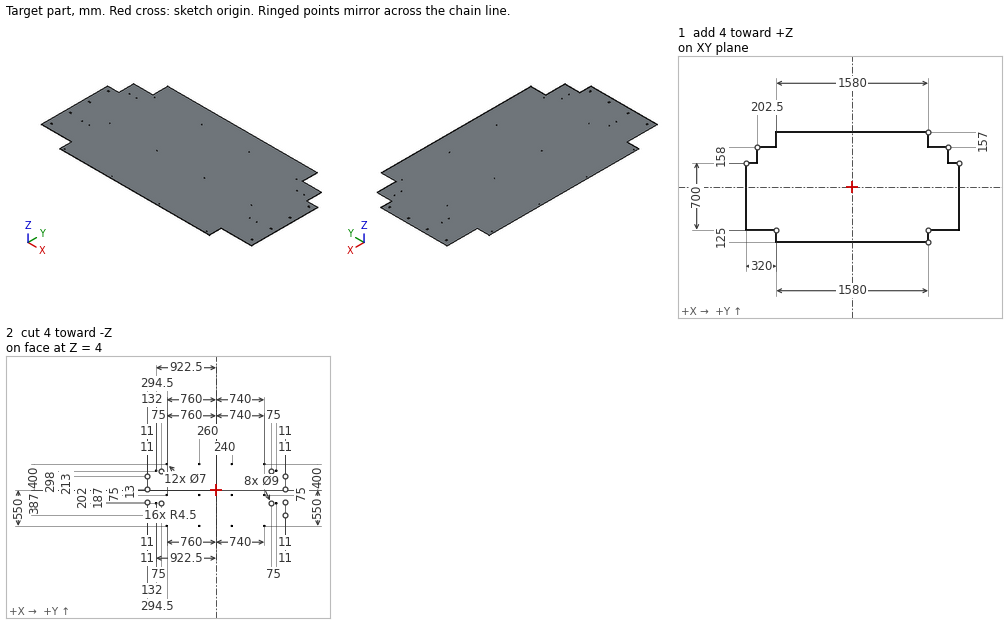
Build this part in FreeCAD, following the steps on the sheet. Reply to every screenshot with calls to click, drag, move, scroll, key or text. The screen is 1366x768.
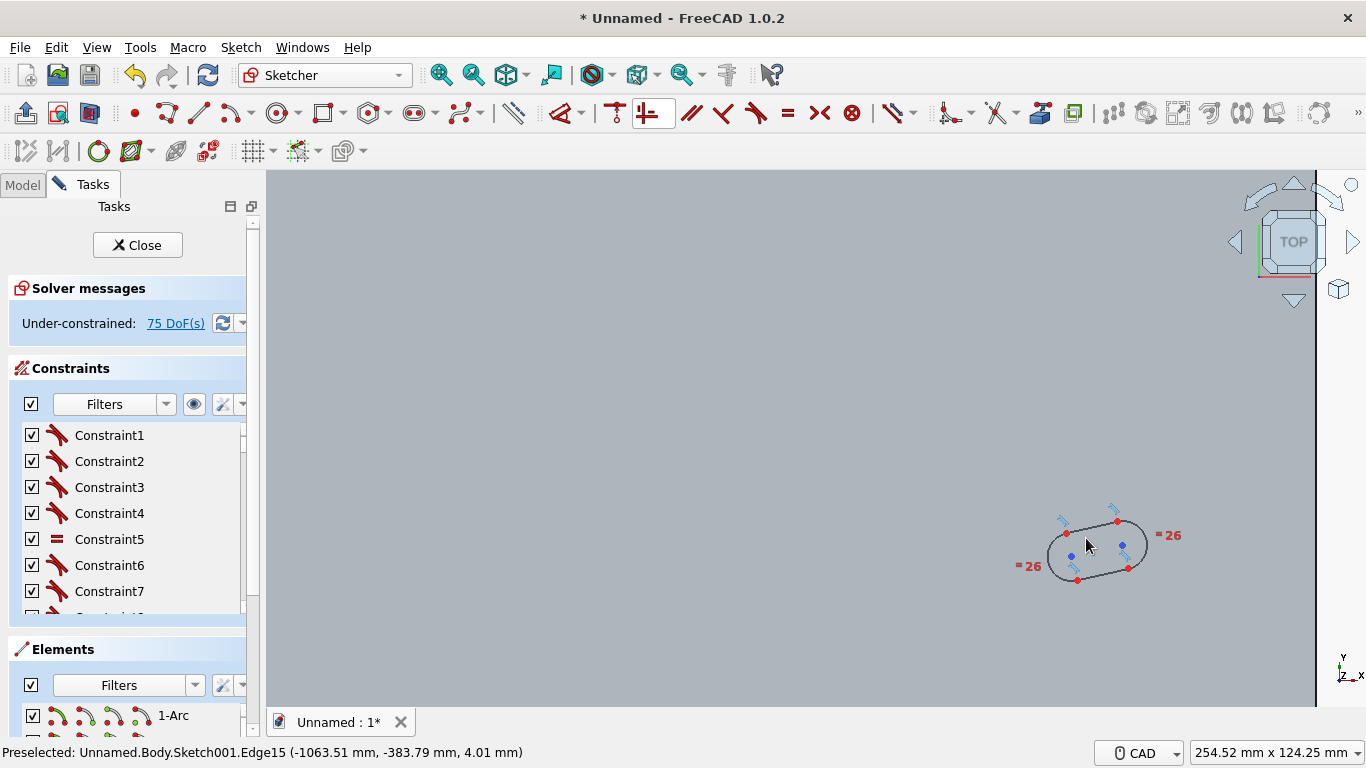
click(1082, 530)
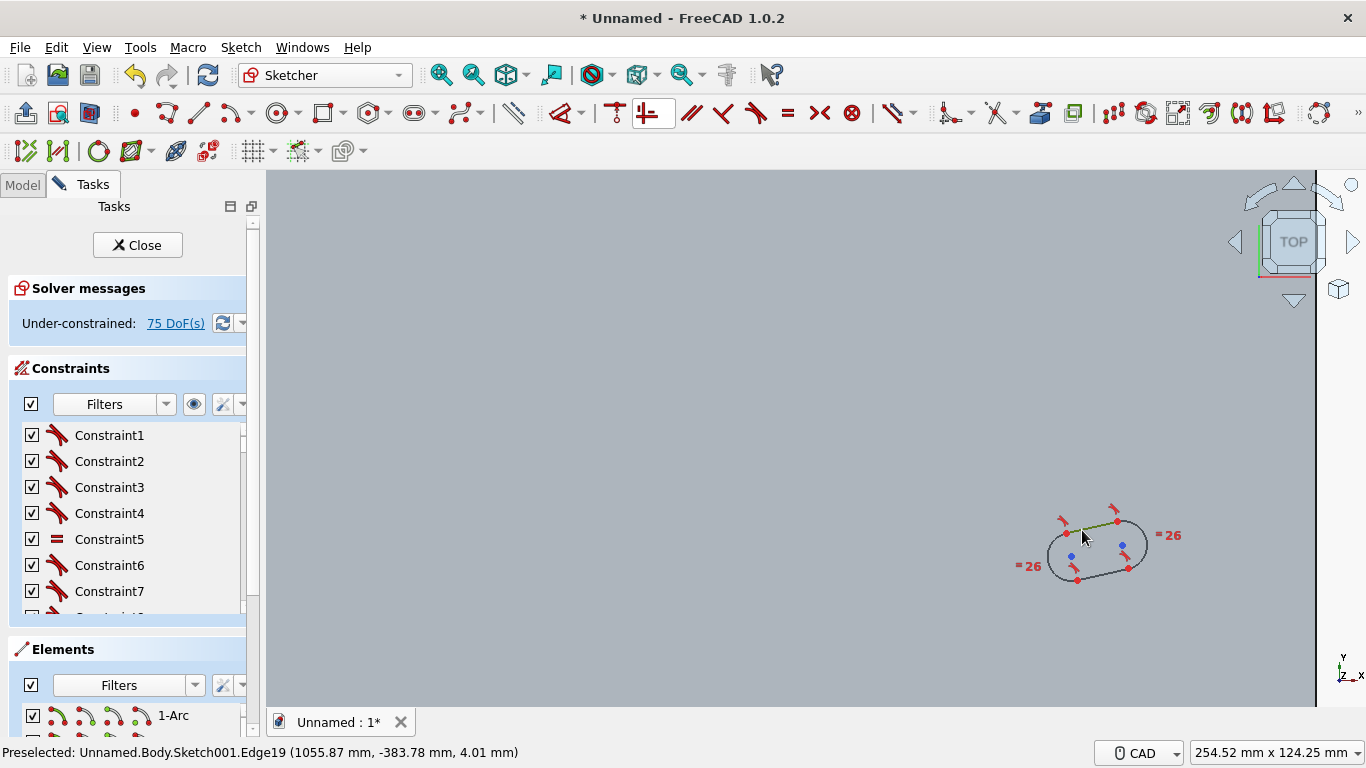
click(670, 114)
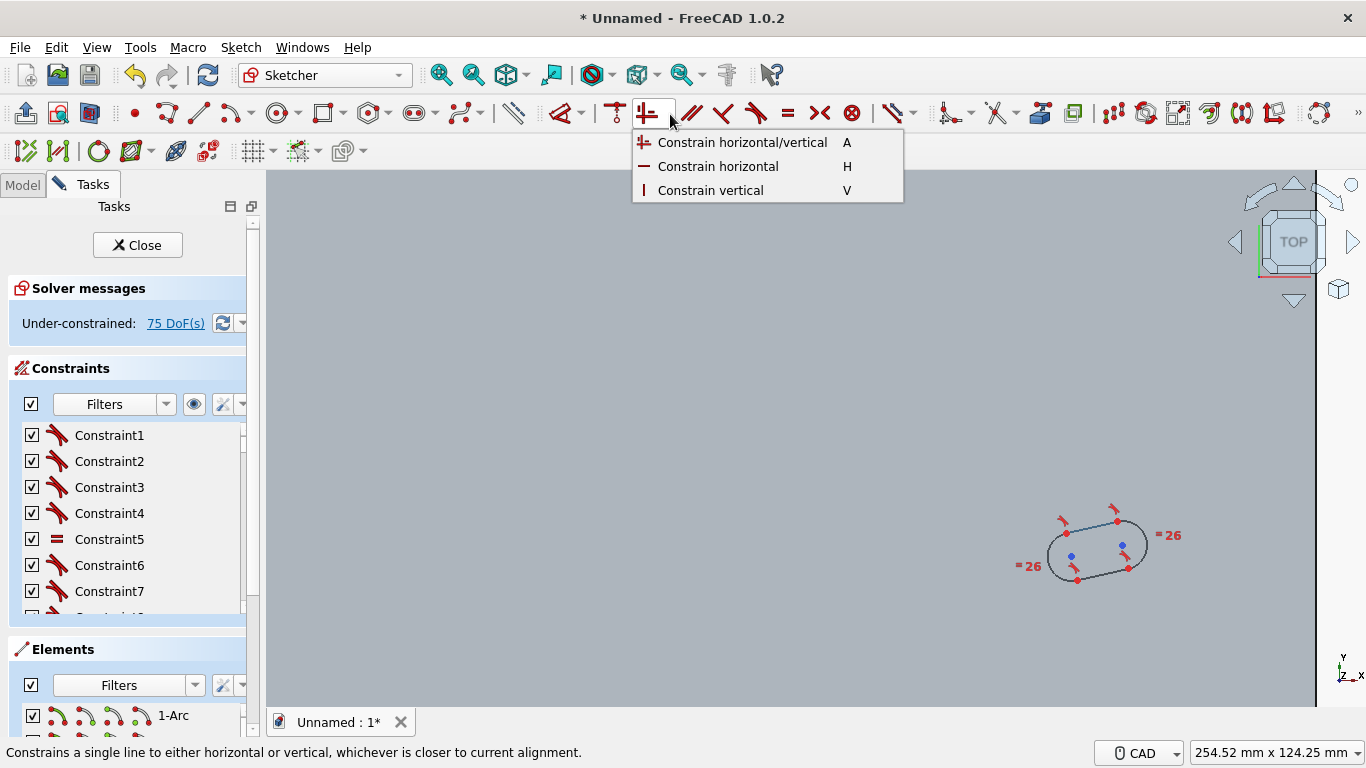
click(768, 166)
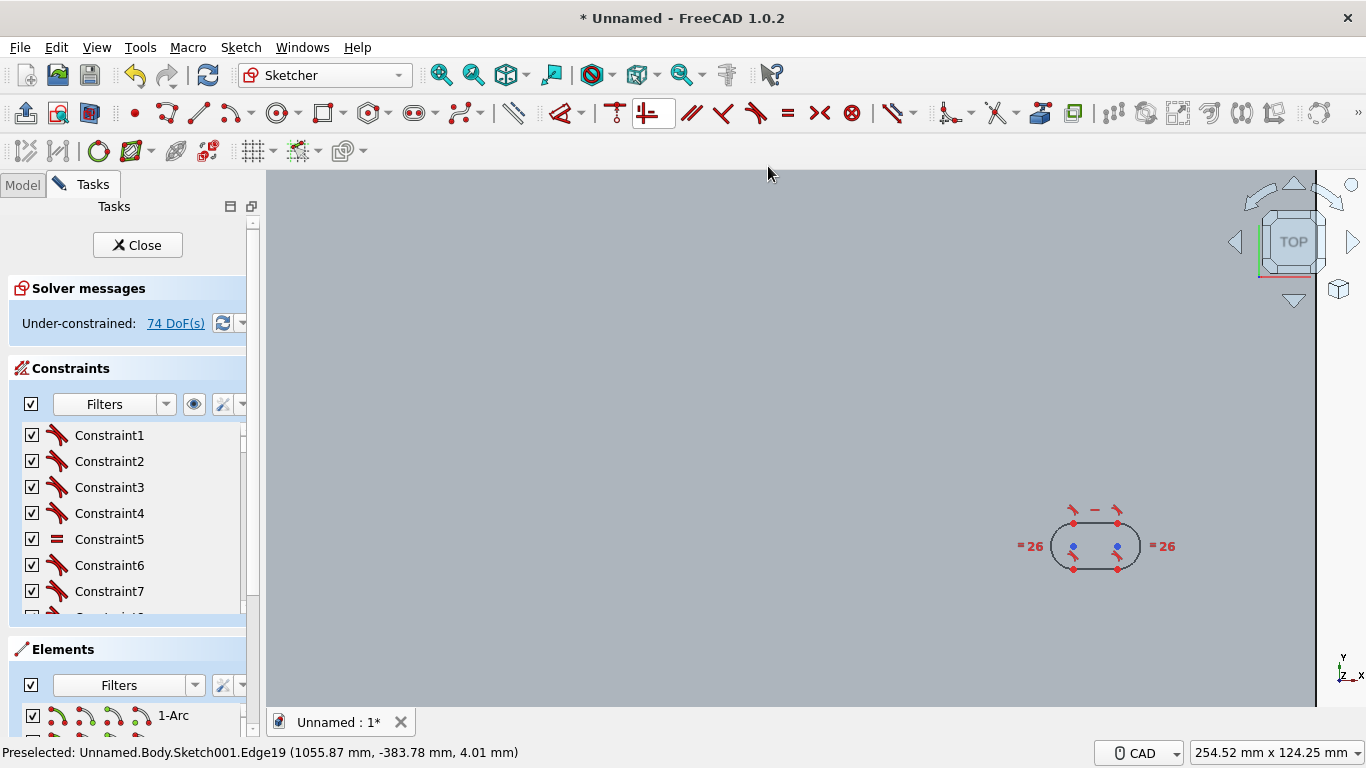
scroll(1087, 538, down, 13)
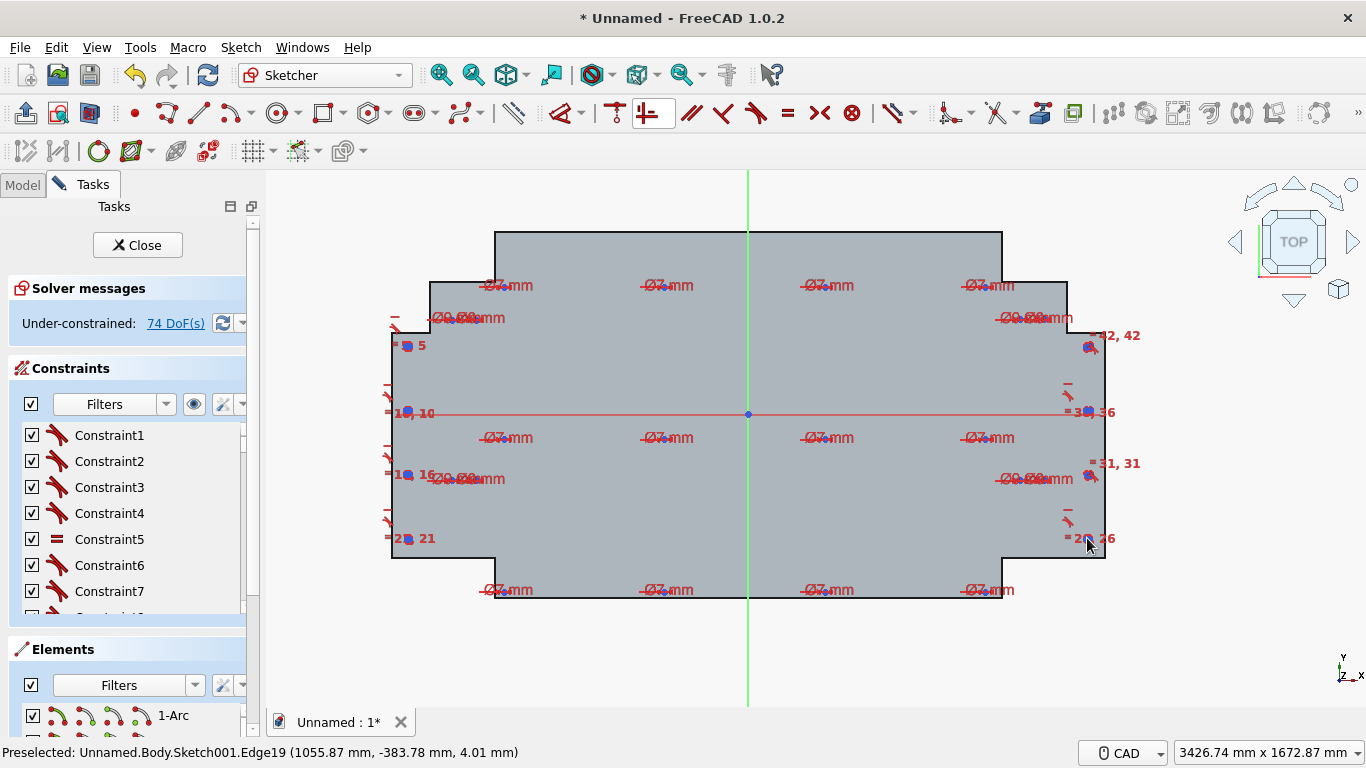
scroll(1088, 474, up, 13)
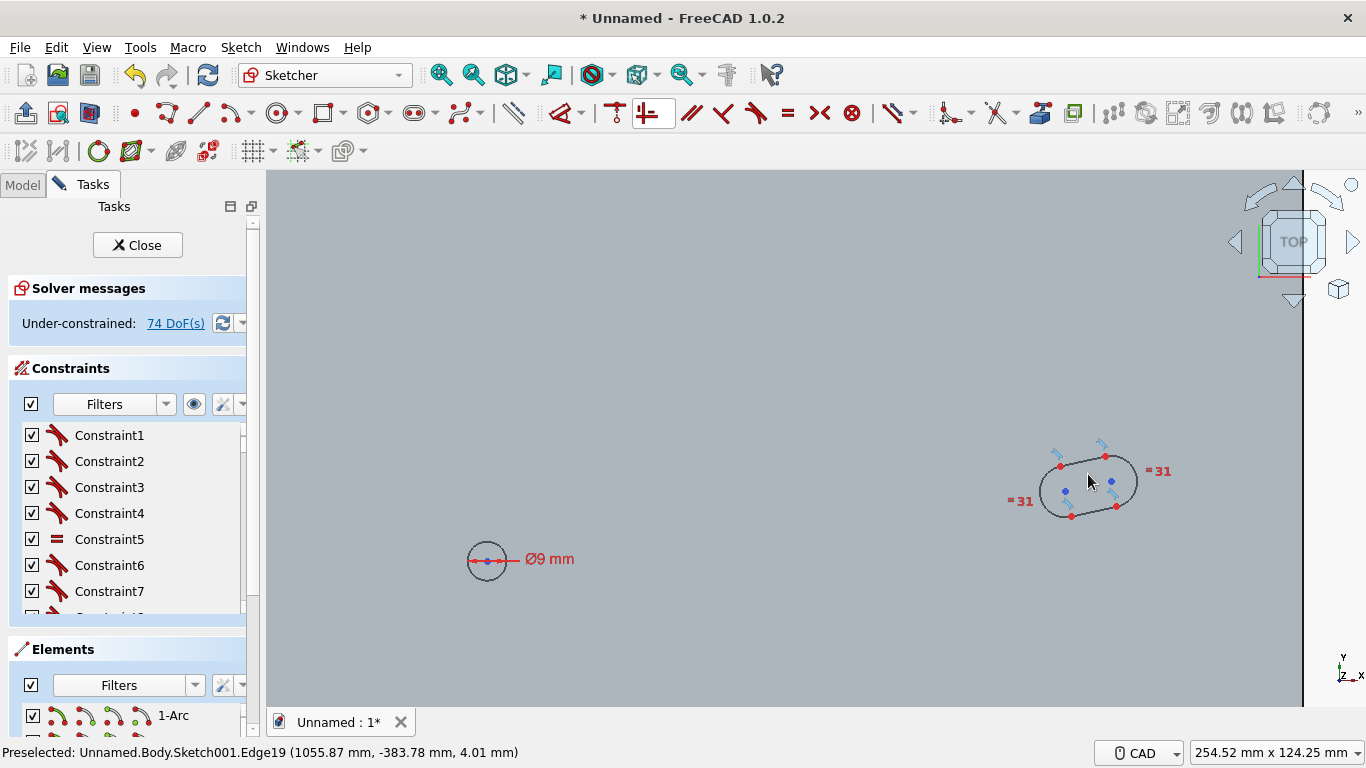
click(1074, 464)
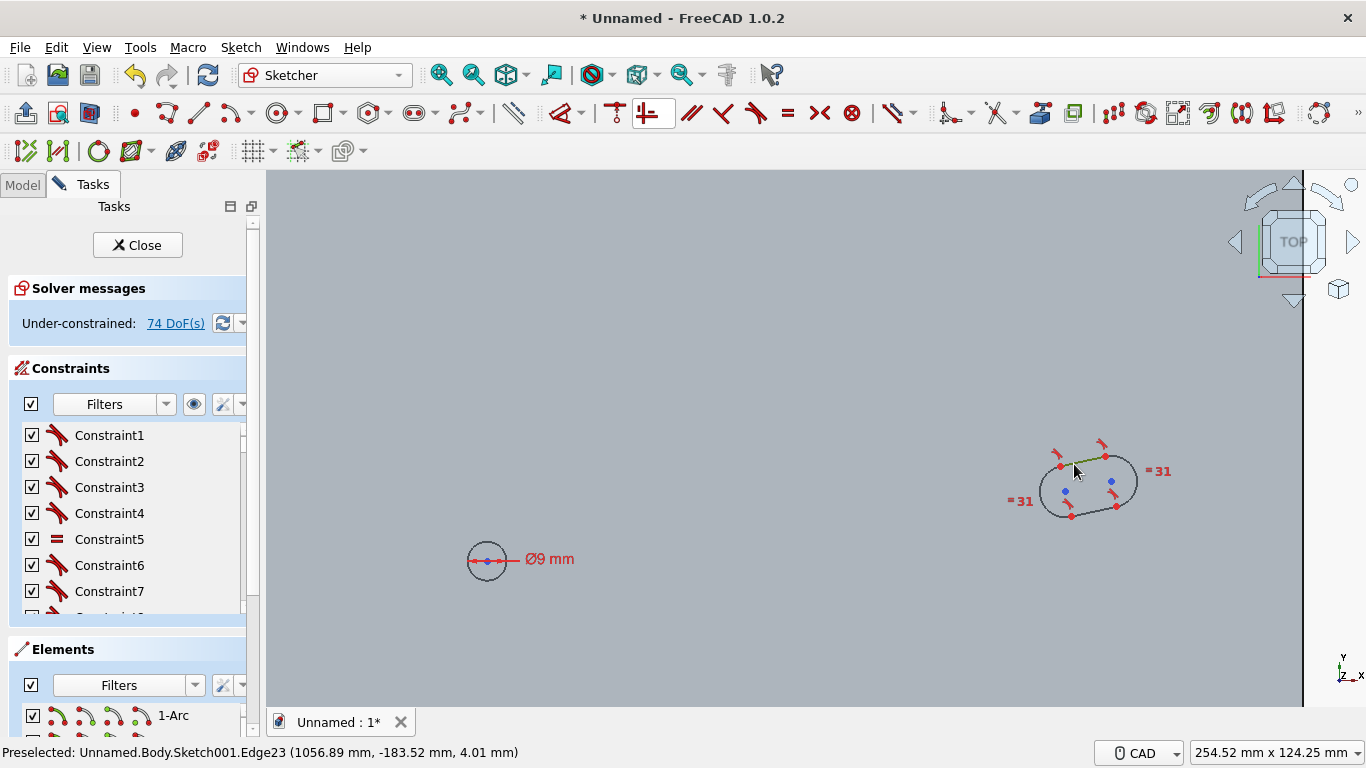
key(h)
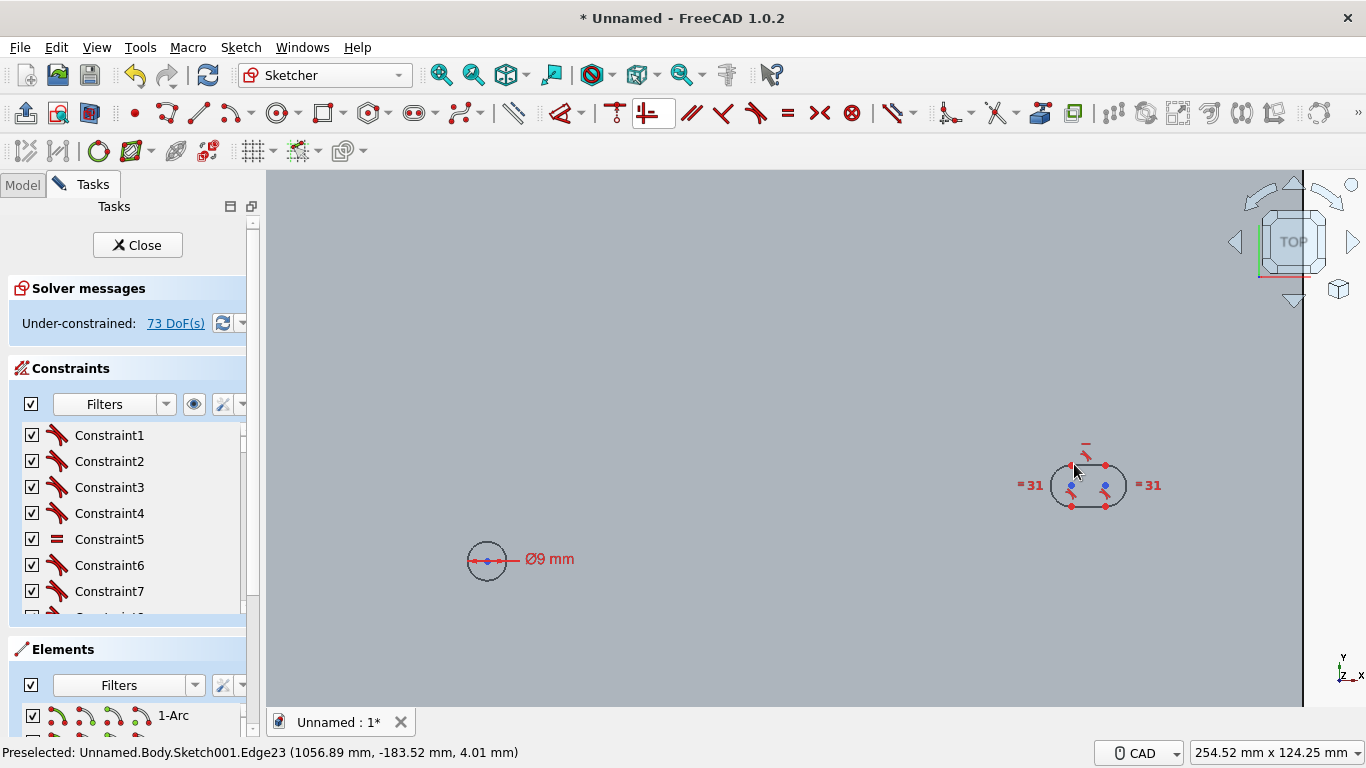
scroll(1088, 474, down, 13)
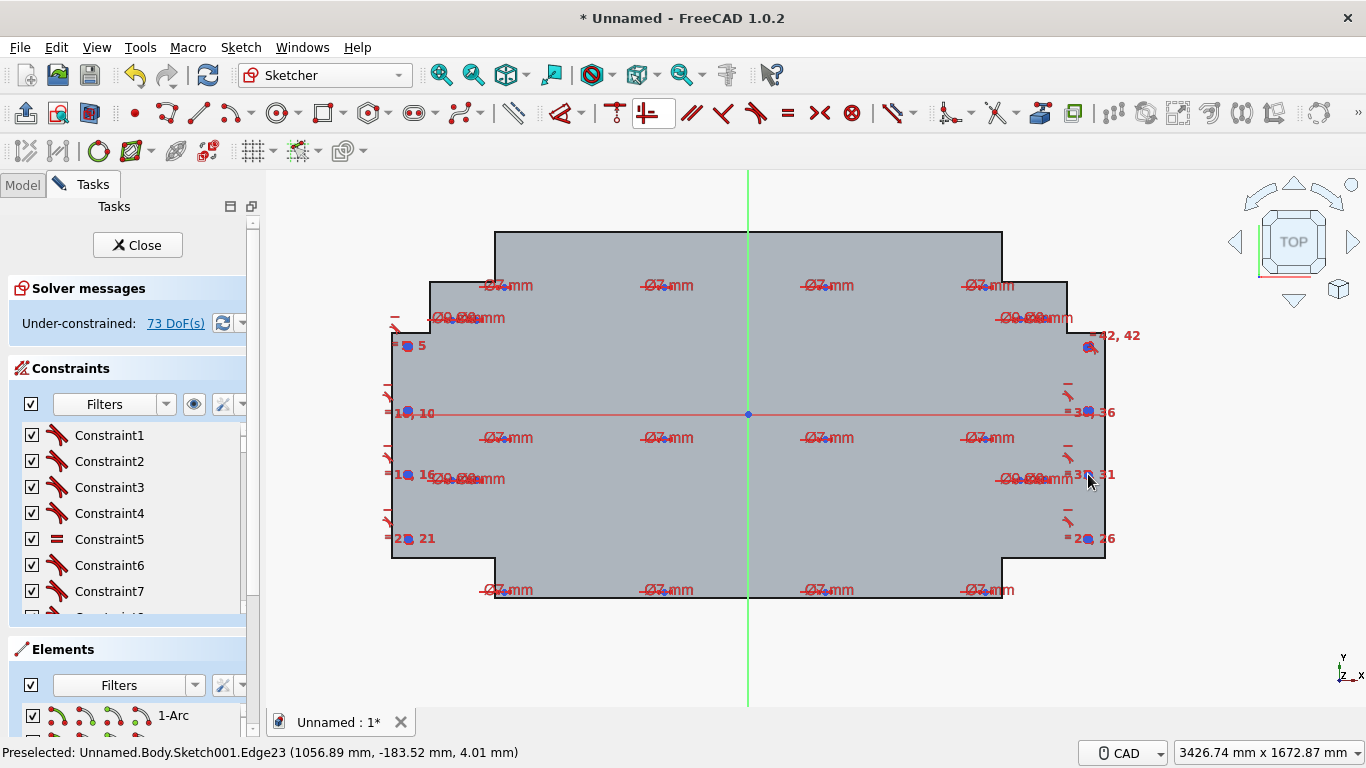
scroll(1087, 345, up, 13)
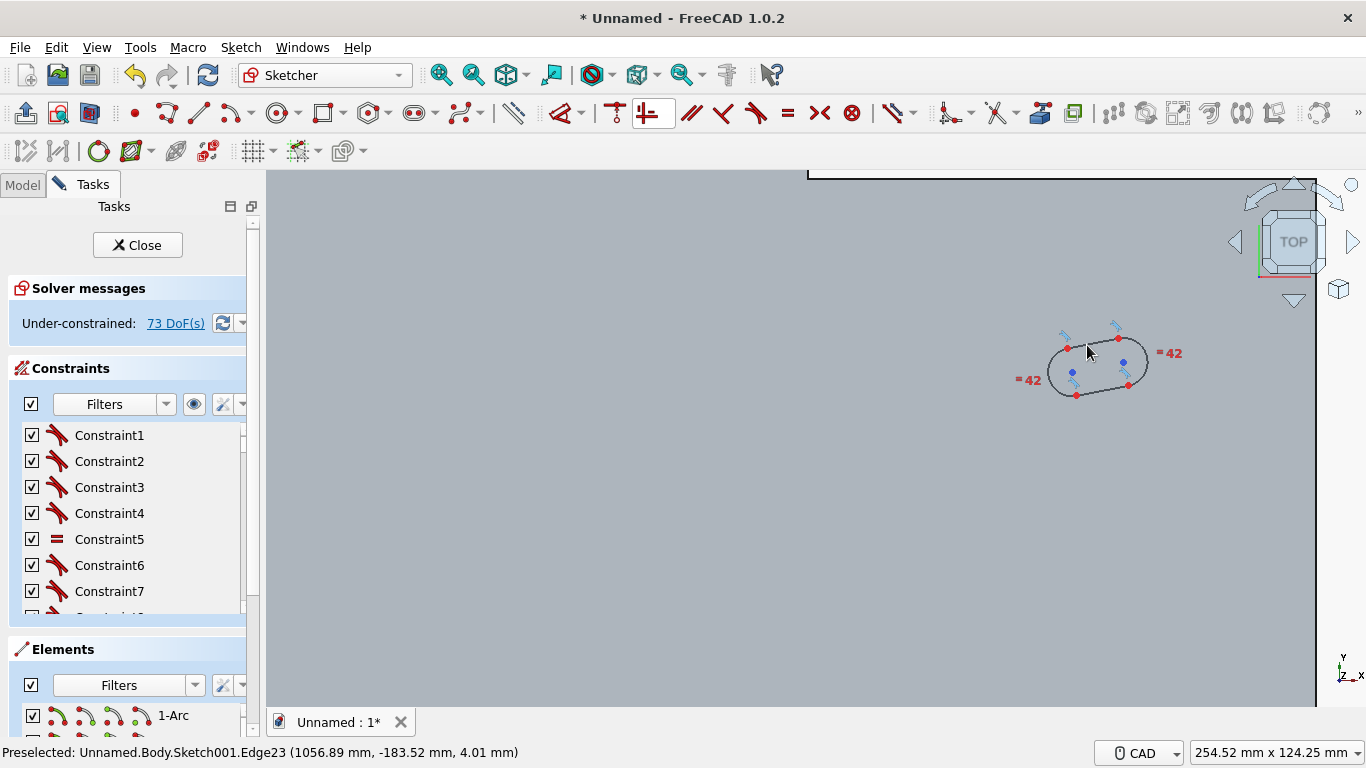
click(1083, 345)